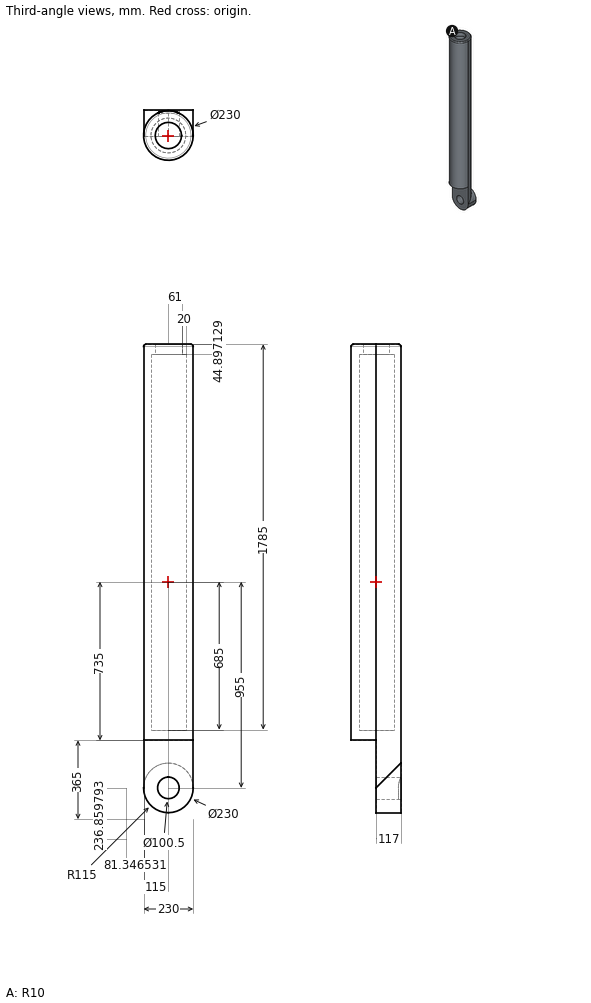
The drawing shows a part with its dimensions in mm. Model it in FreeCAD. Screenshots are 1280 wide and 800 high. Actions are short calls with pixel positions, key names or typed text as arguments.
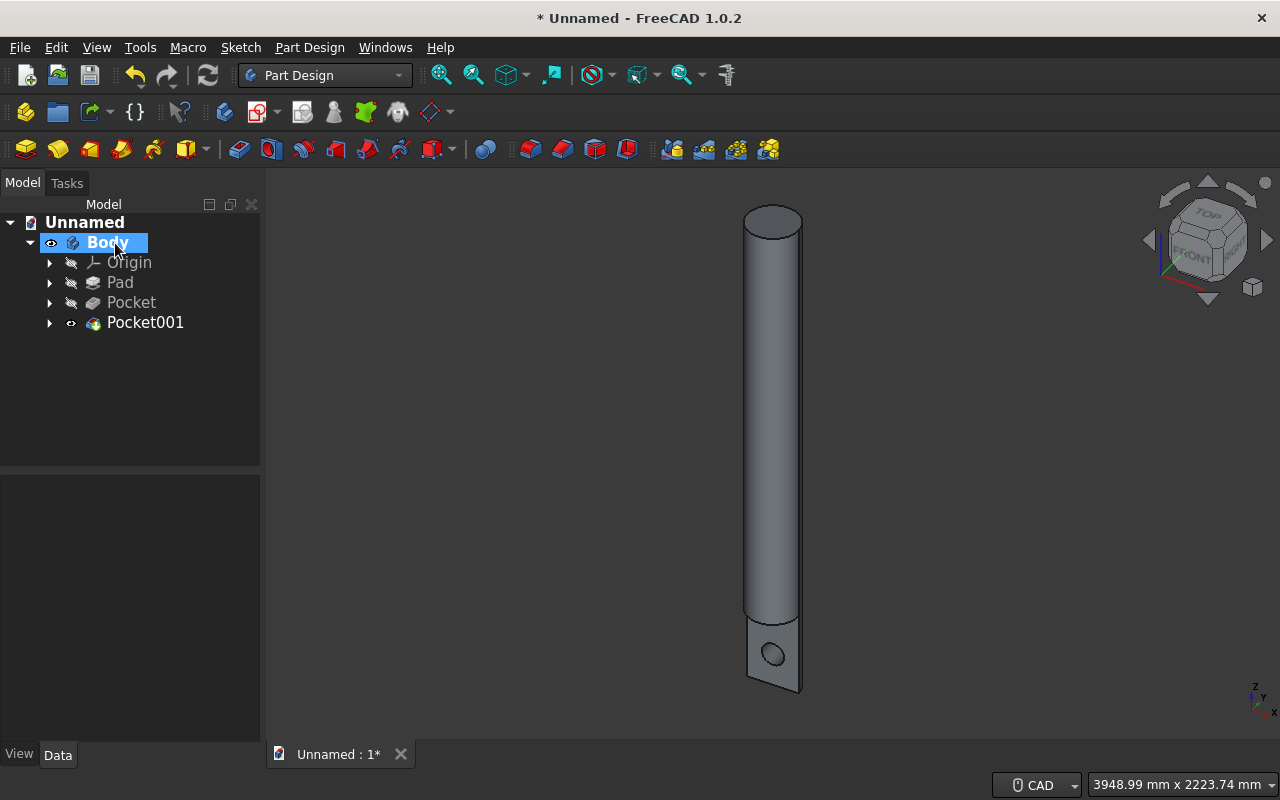
click(258, 112)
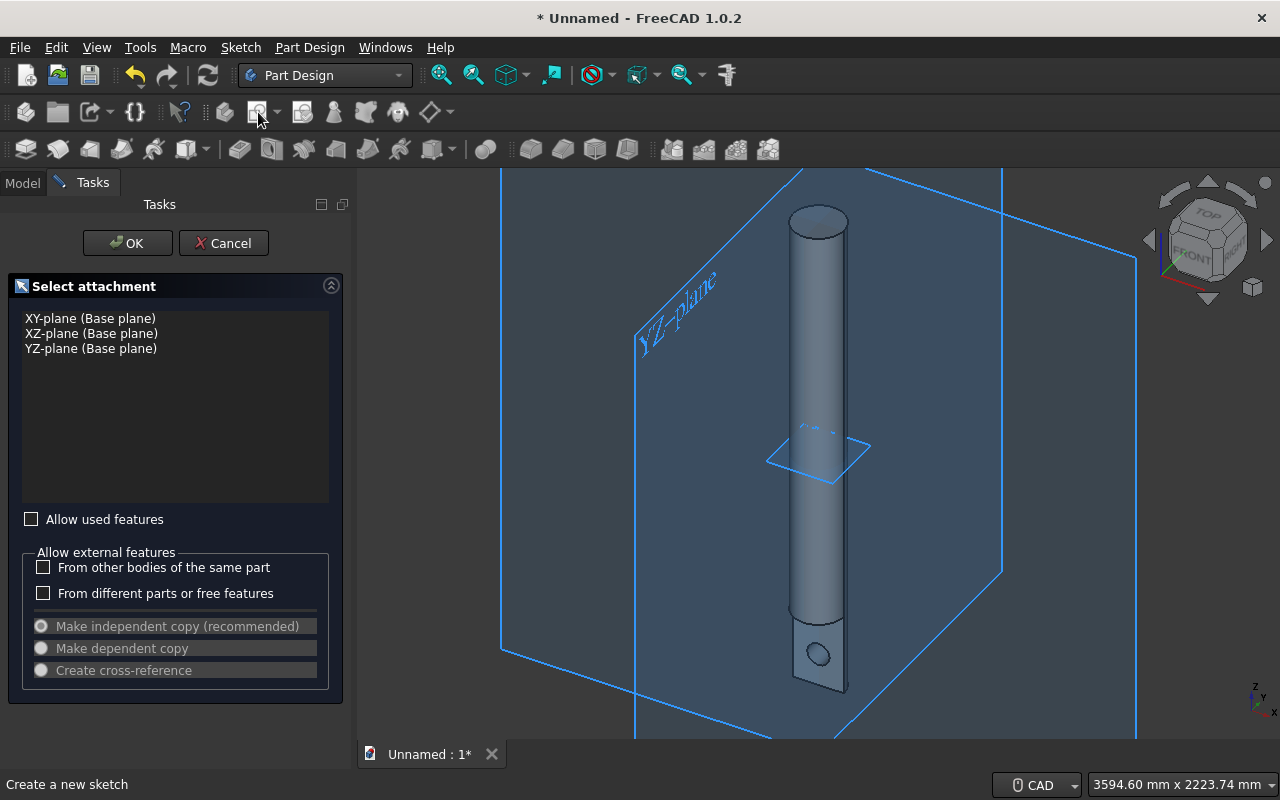
click(82, 334)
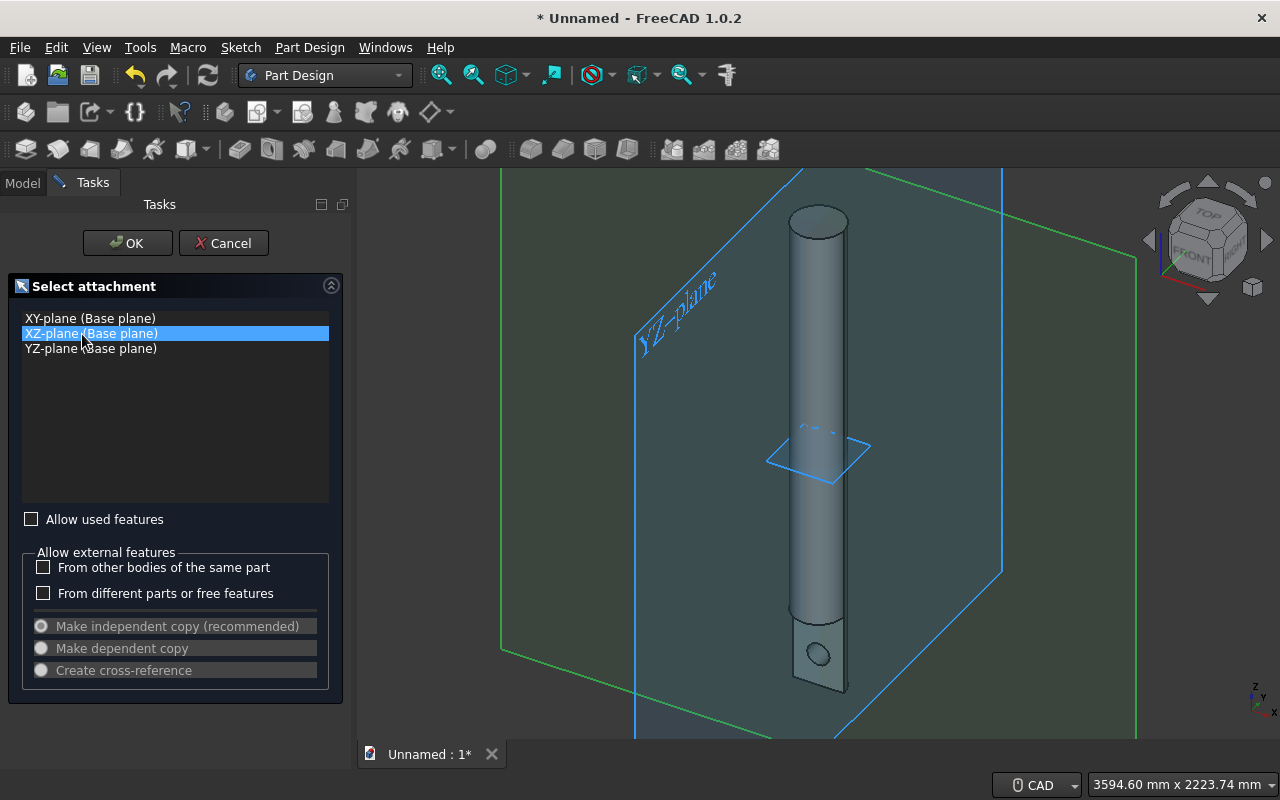
click(128, 243)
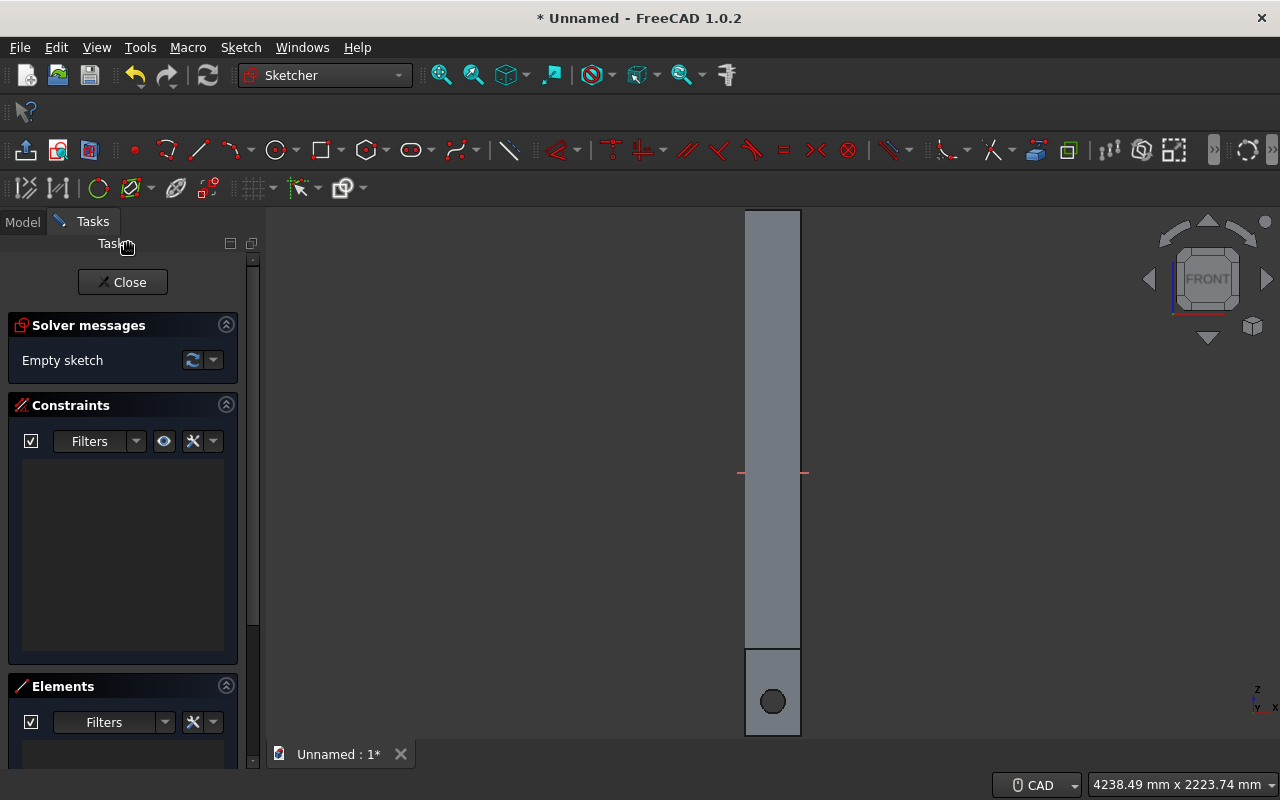
click(90, 150)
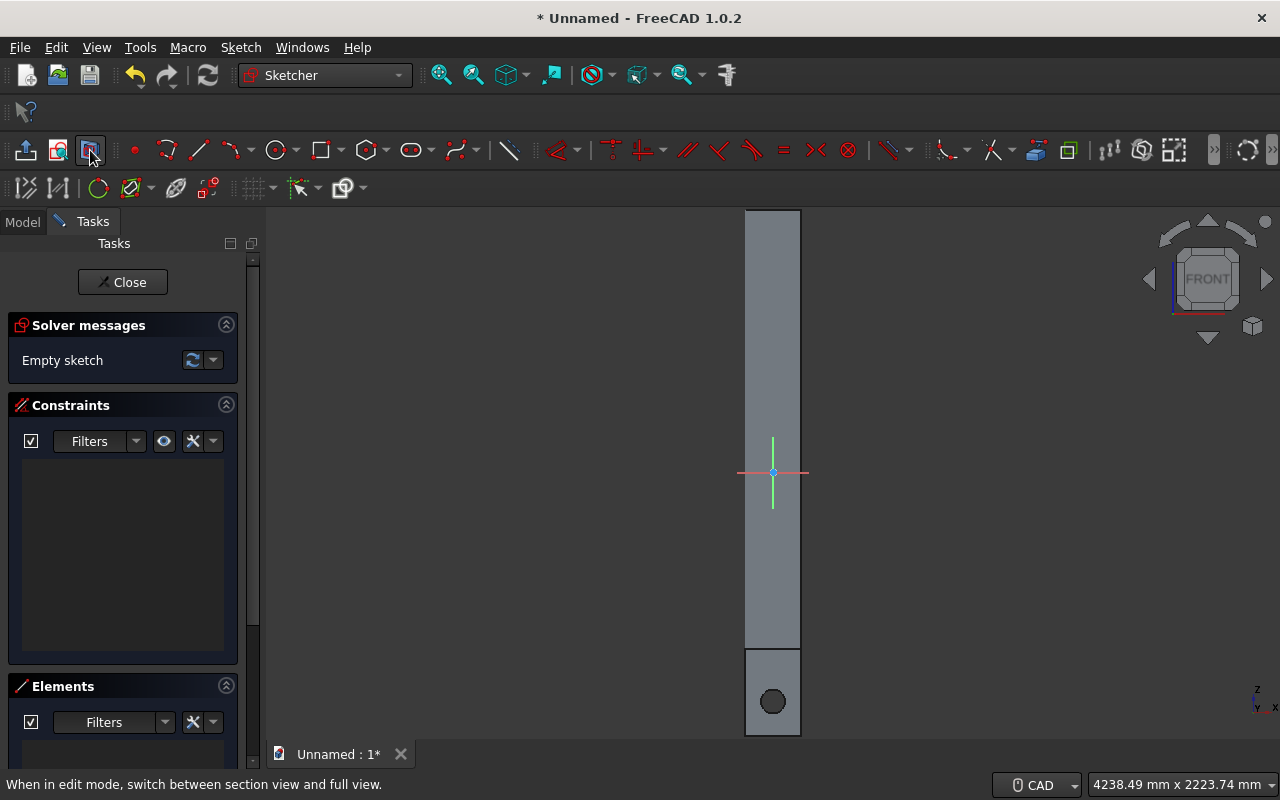
scroll(704, 473, down, 5)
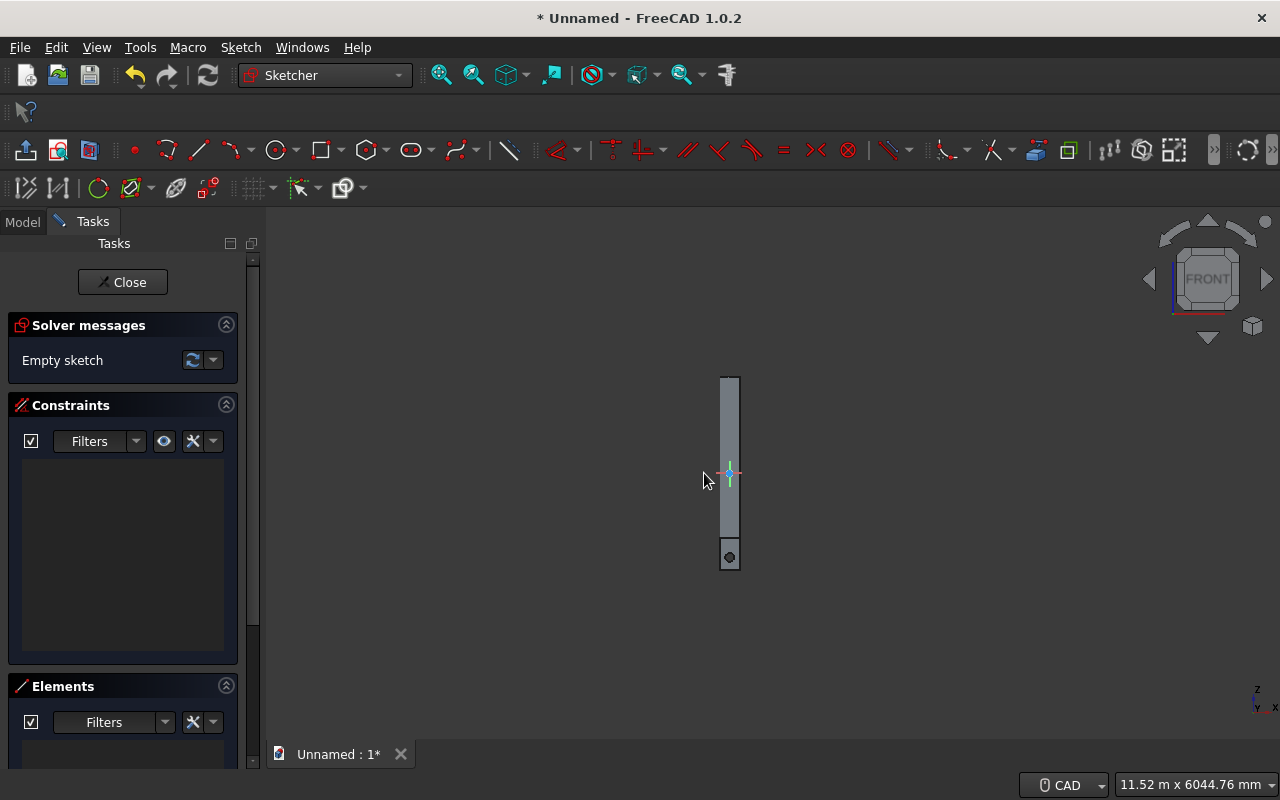
scroll(722, 574, up, 14)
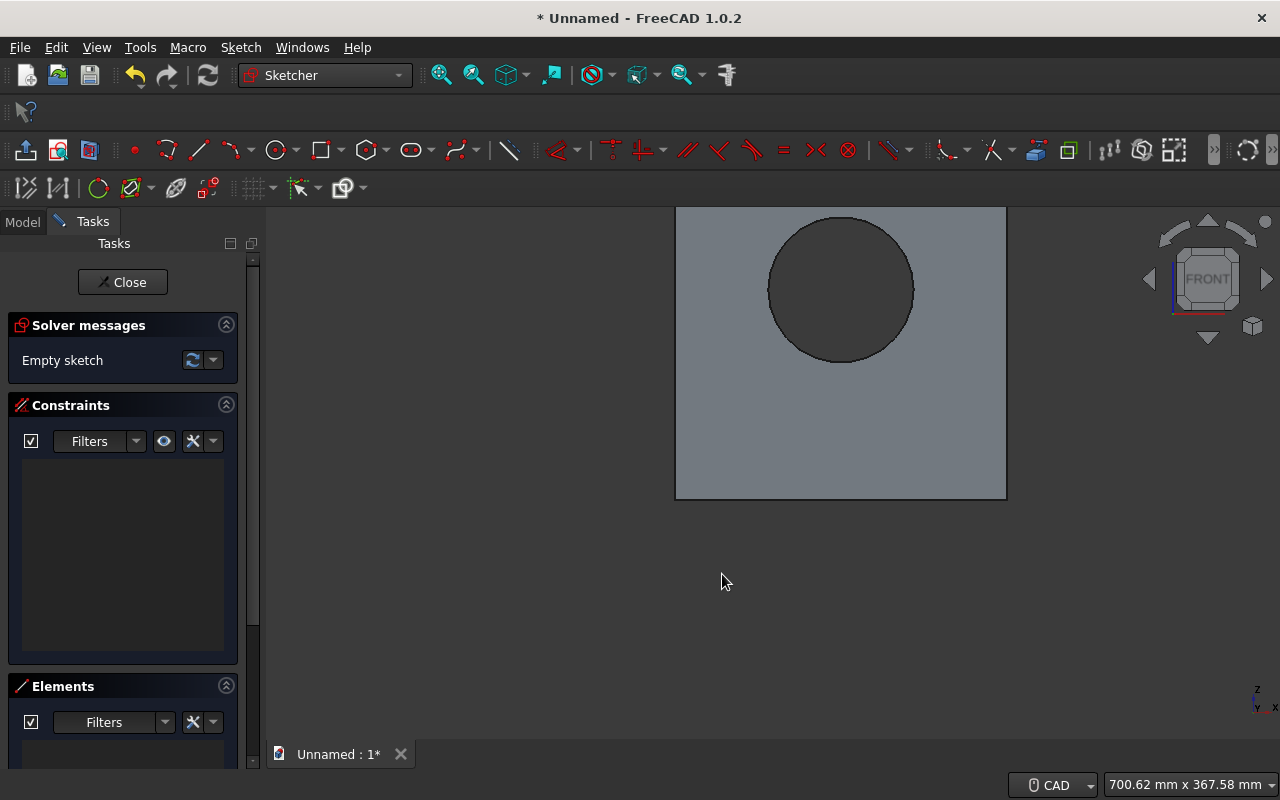
click(168, 150)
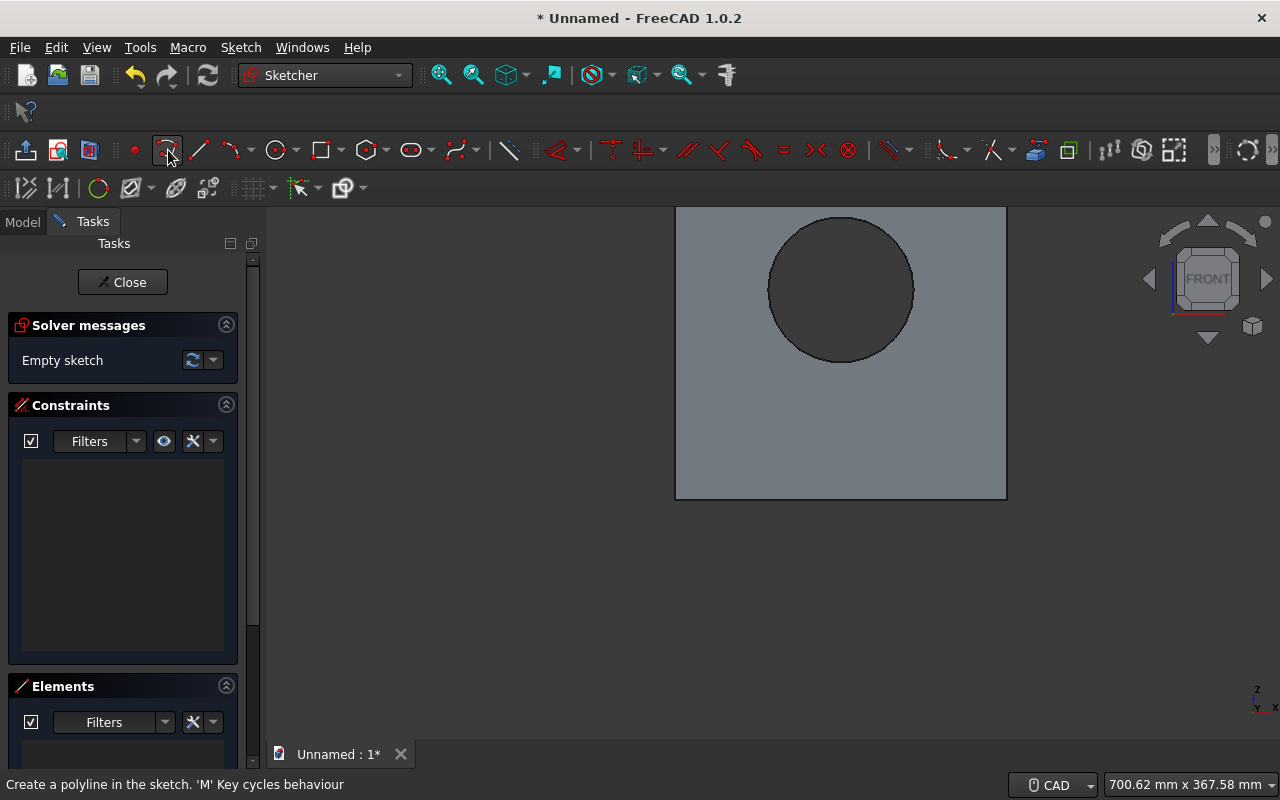
click(675, 290)
click(557, 290)
click(557, 633)
click(841, 633)
click(832, 456)
right_click(832, 456)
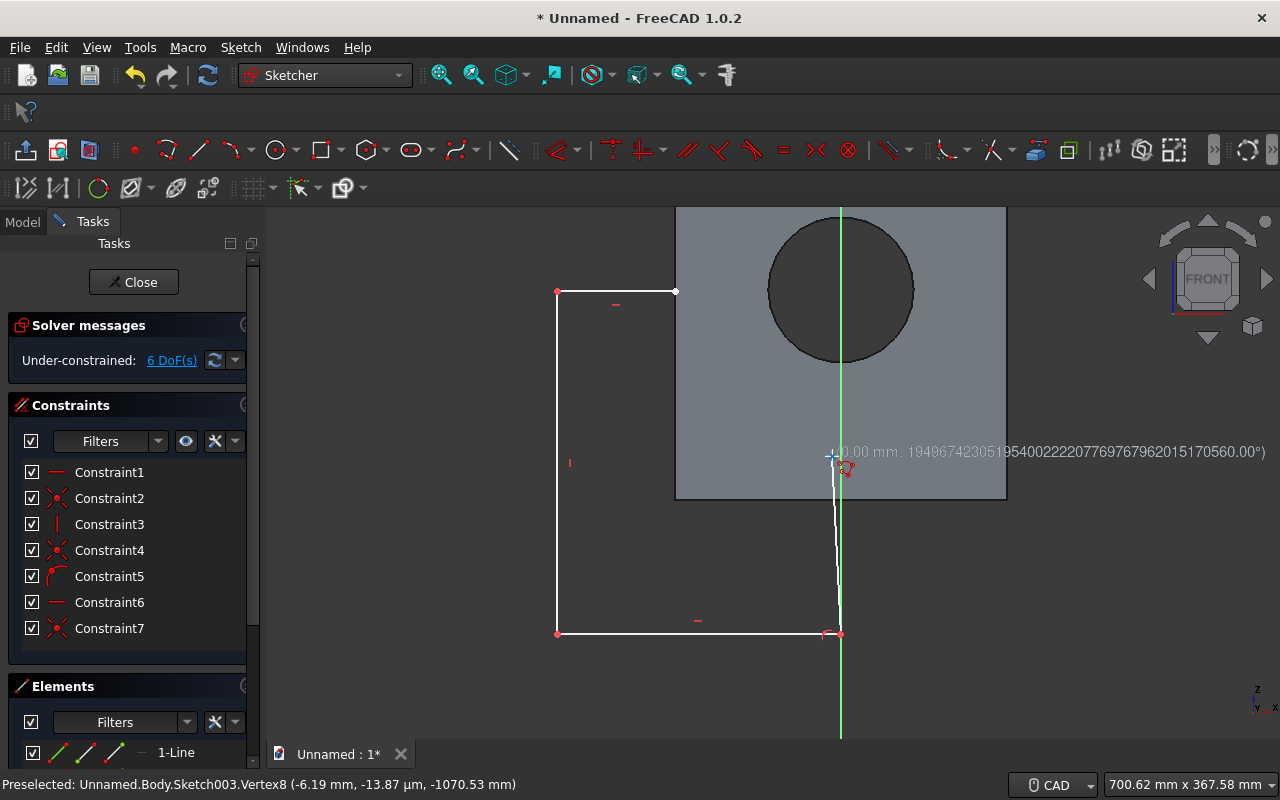
click(232, 150)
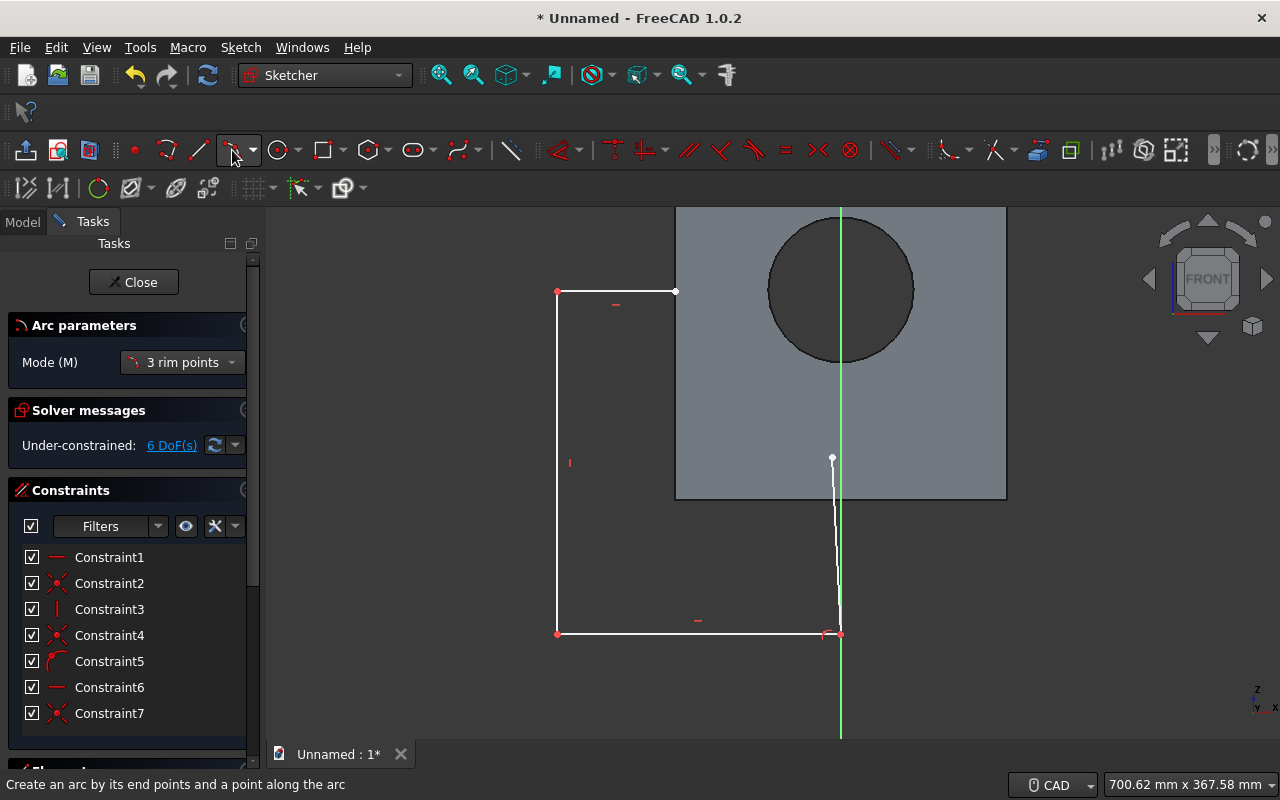
click(832, 457)
click(675, 291)
click(723, 407)
key(Escape)